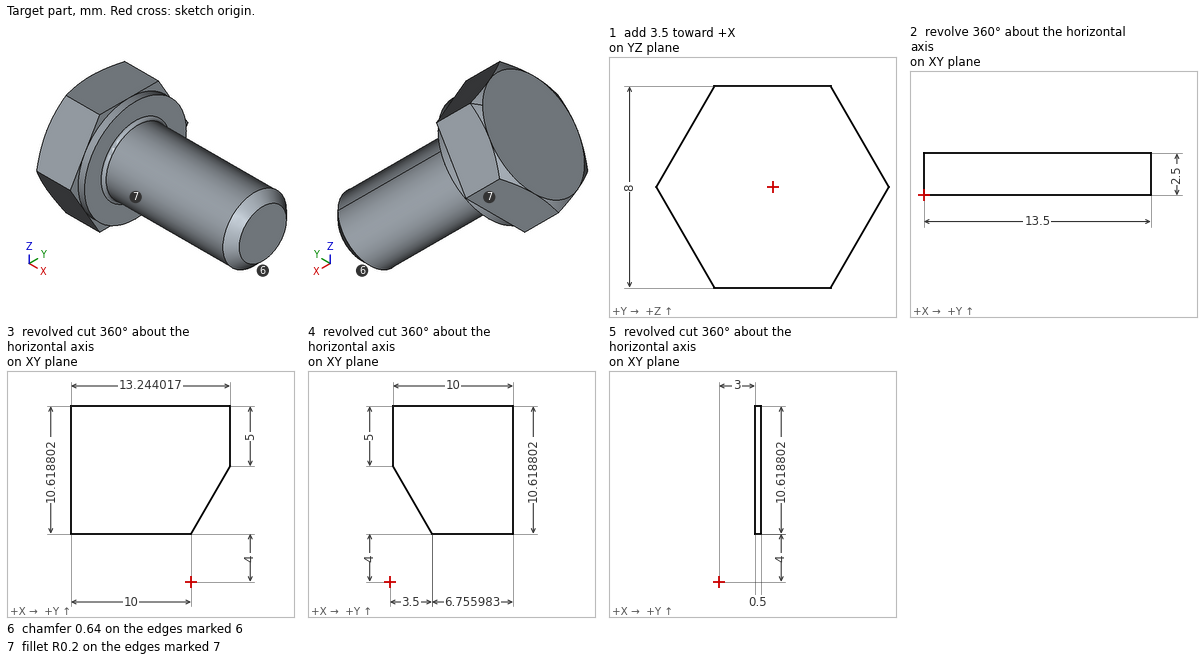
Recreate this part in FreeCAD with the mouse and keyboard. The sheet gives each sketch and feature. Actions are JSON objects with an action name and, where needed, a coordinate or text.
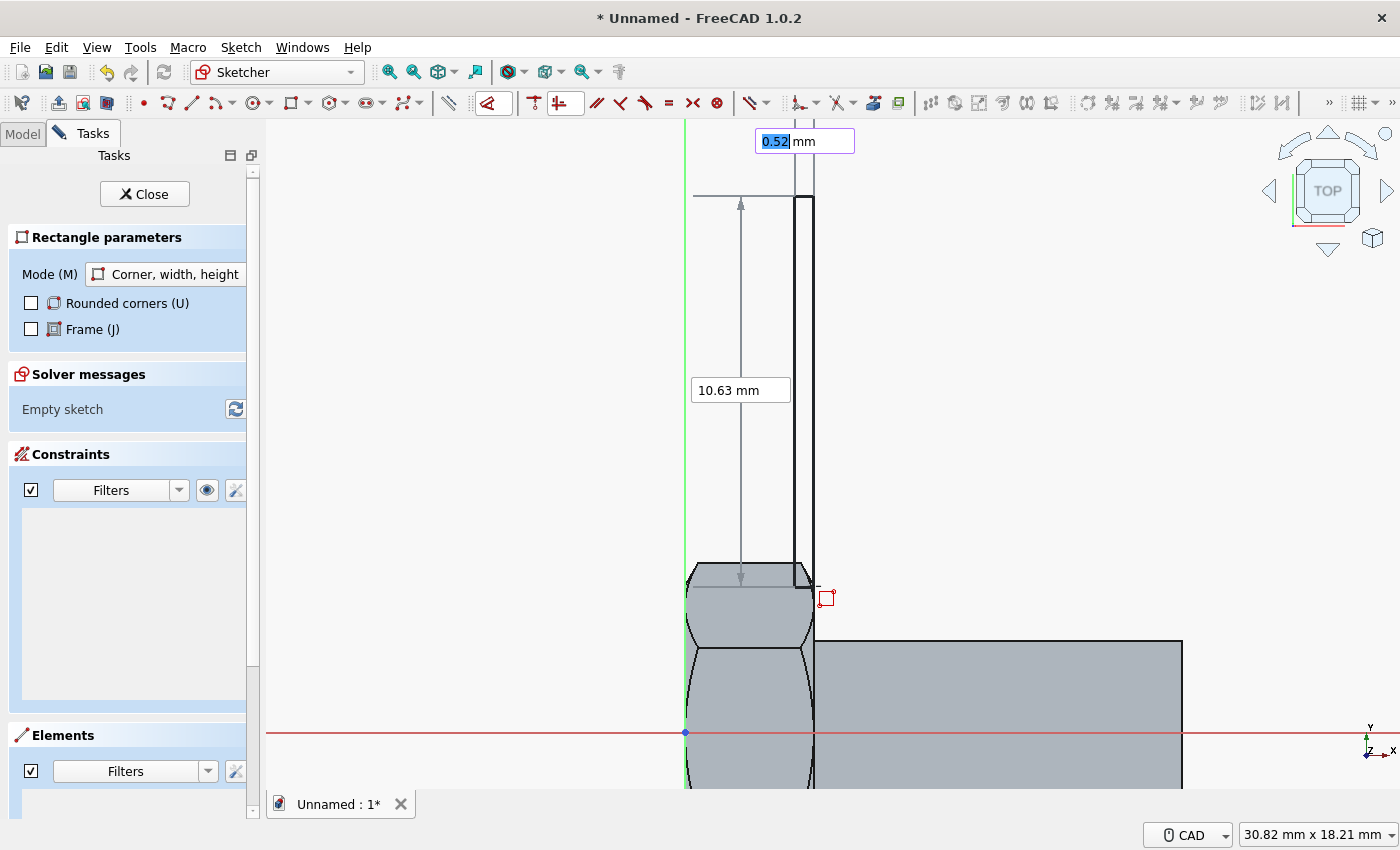
{"action": "type", "text": "0.5"}
{"action": "key", "text": "Tab"}
{"action": "type", "text": "10.618802"}
{"action": "key", "text": "Return"}
{"action": "key", "text": "Escape"}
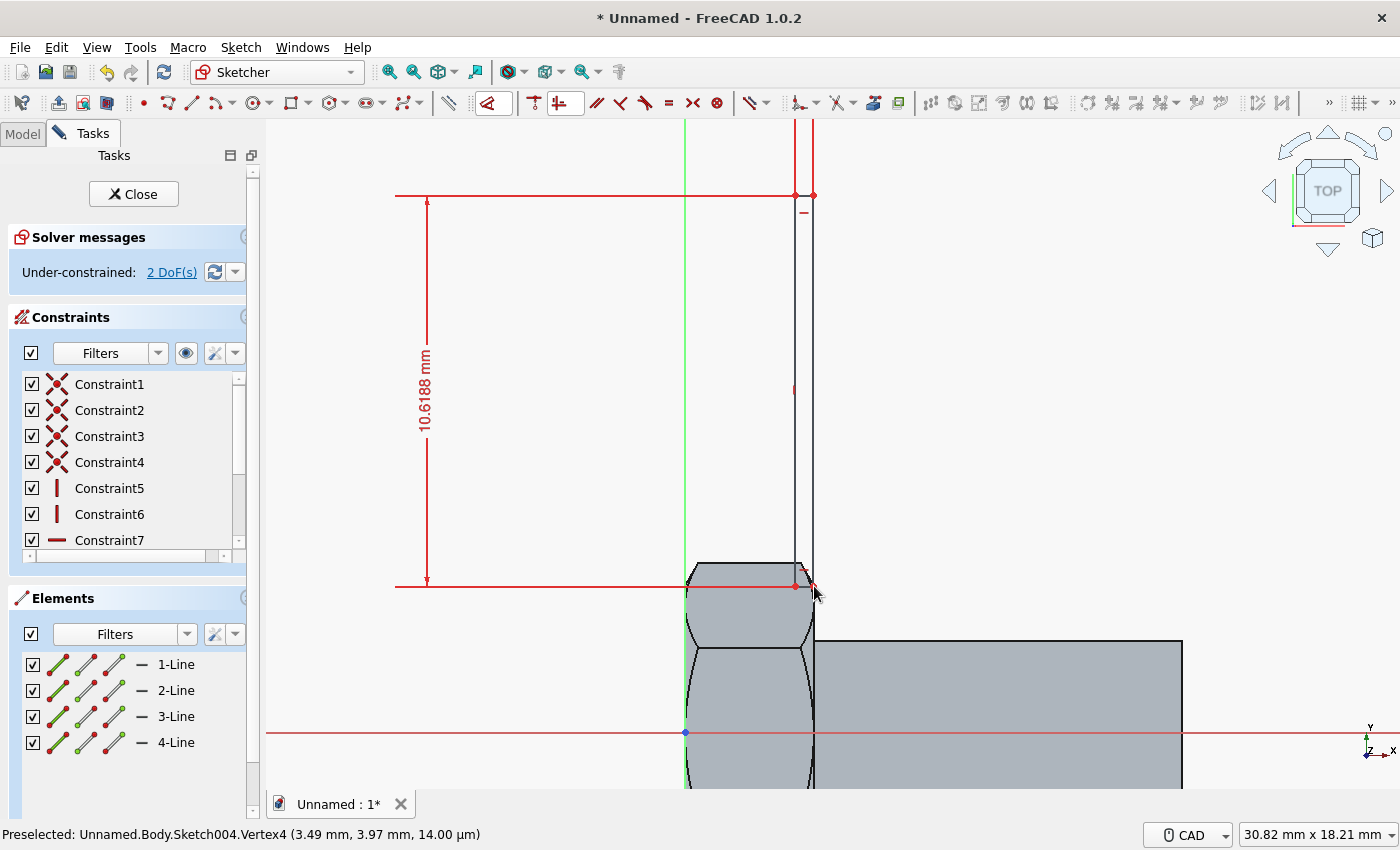
{"action": "left_click", "coordinate": [795, 196]}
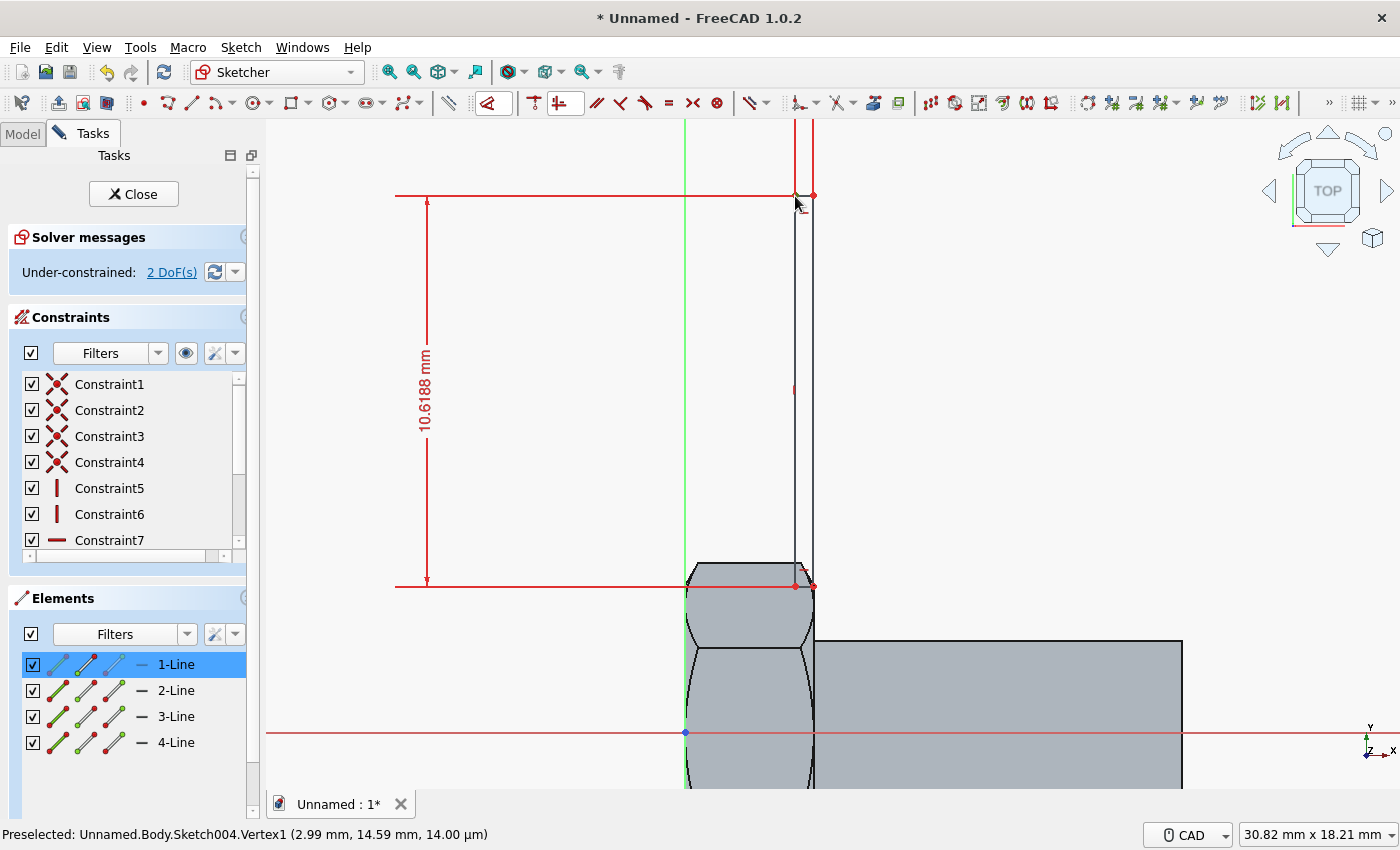
{"action": "key", "text": "l"}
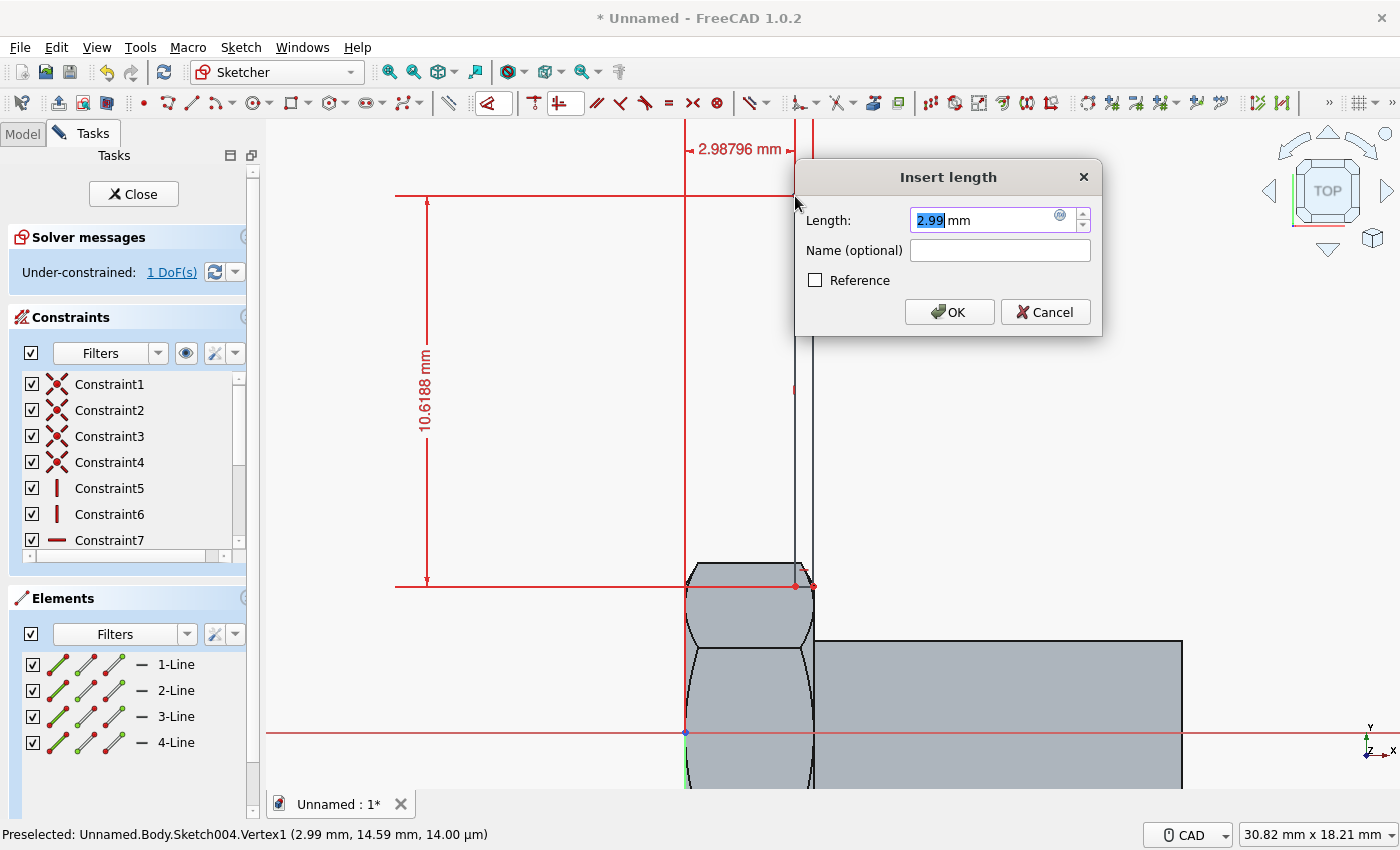
{"action": "type", "text": "3"}
{"action": "key", "text": "Return"}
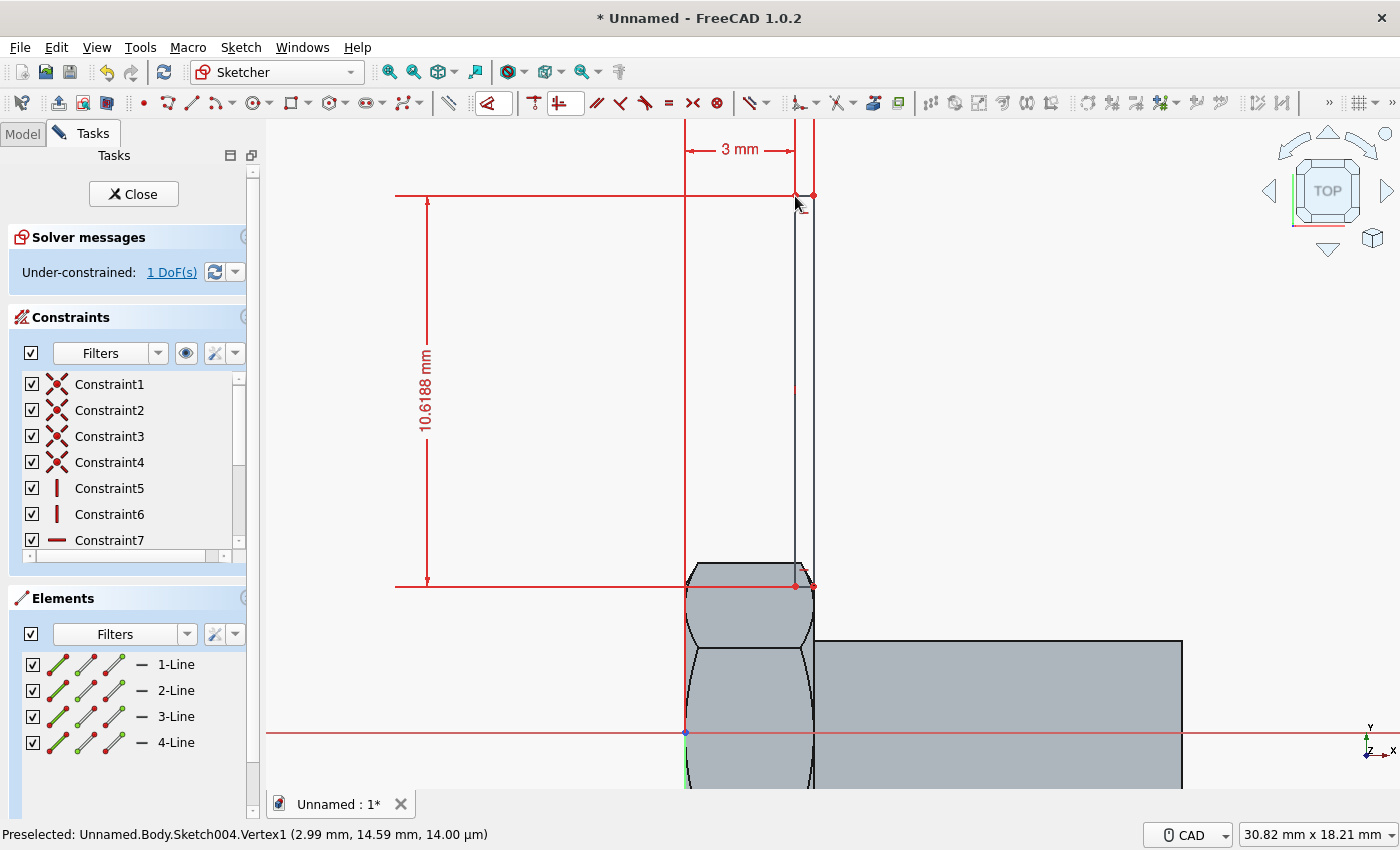
{"action": "left_click", "coordinate": [795, 587]}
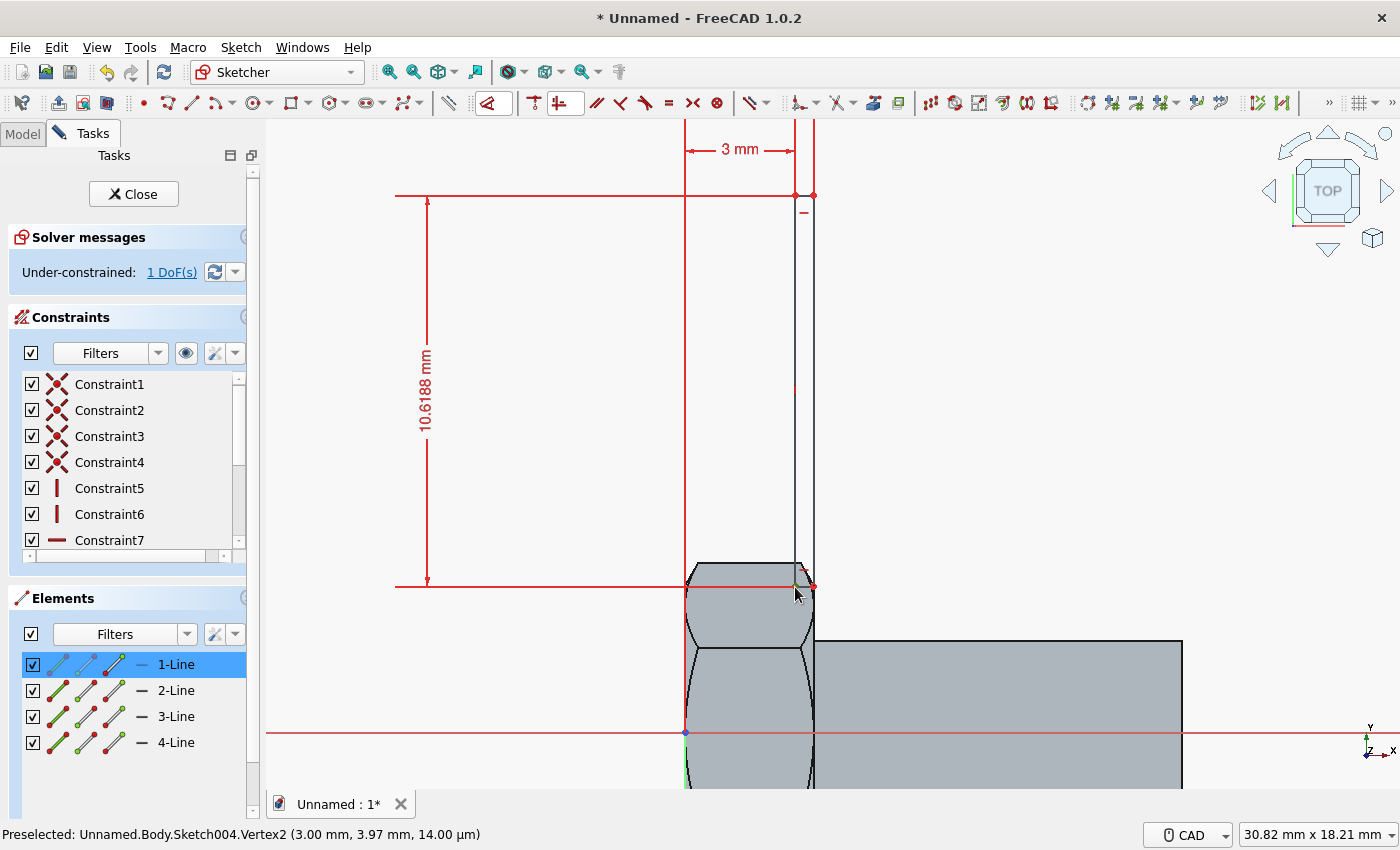
{"action": "key", "text": "i"}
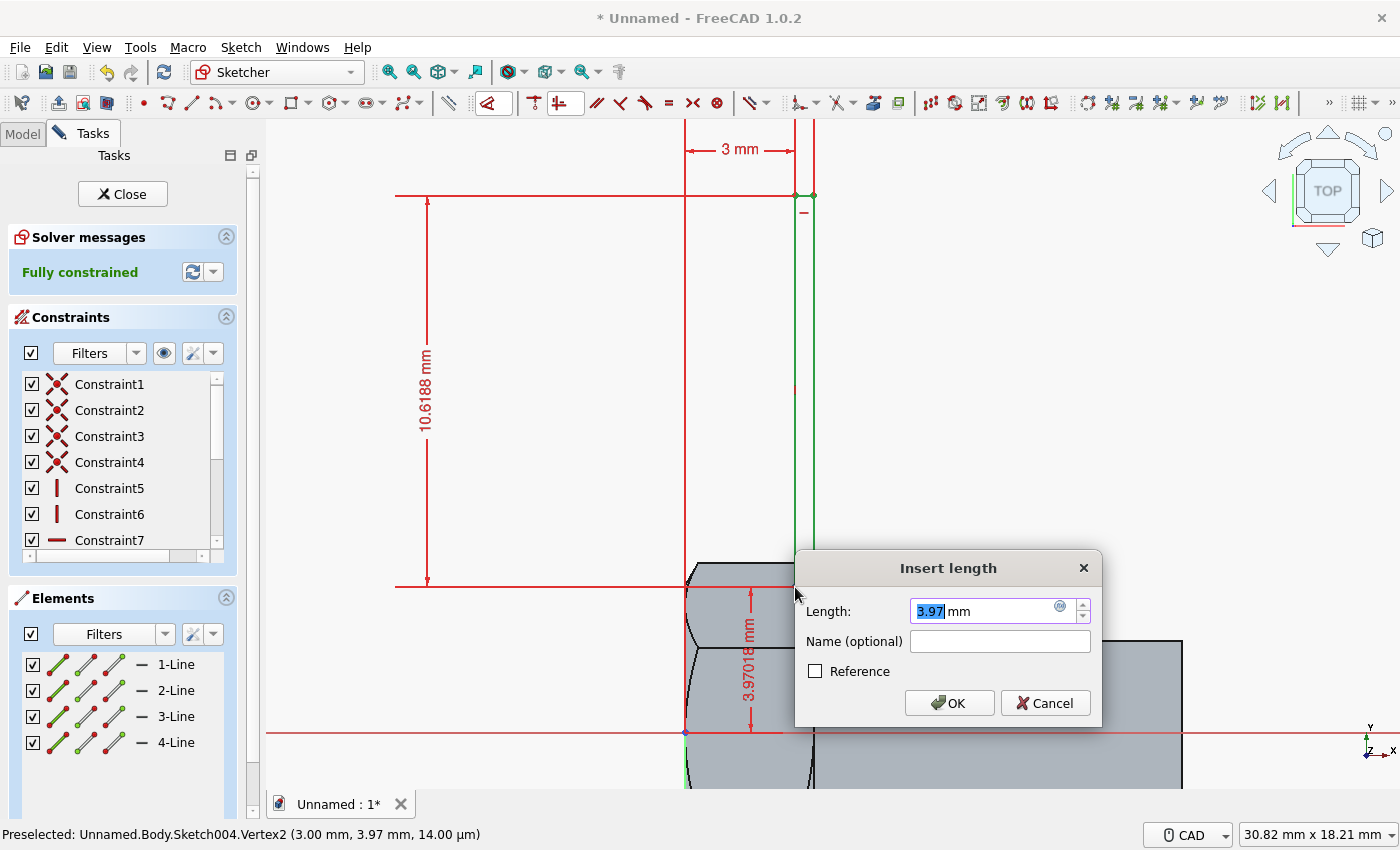
{"action": "type", "text": "4"}
{"action": "key", "text": "Return"}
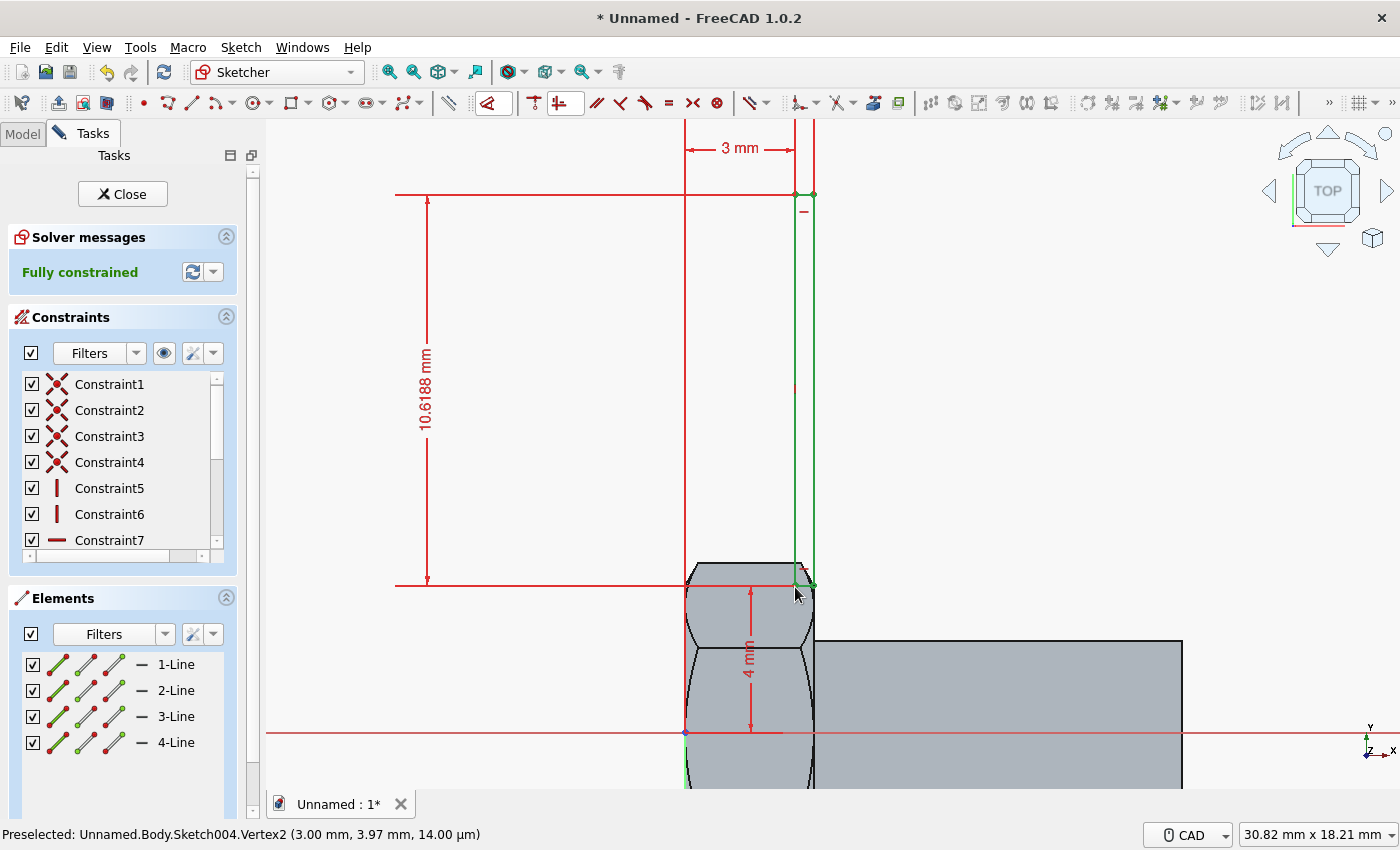
{"action": "left_click", "coordinate": [123, 194]}